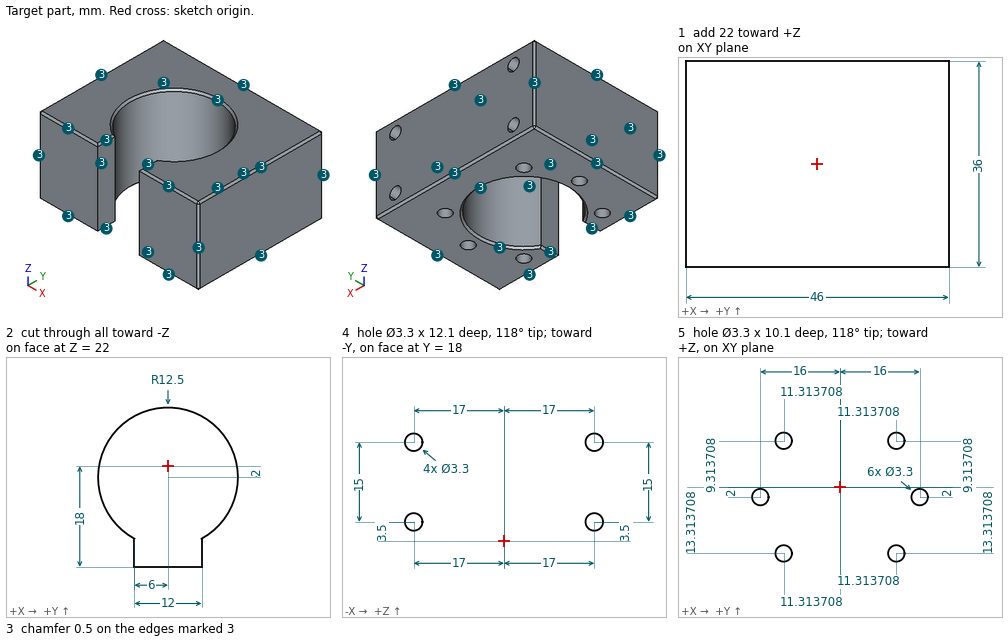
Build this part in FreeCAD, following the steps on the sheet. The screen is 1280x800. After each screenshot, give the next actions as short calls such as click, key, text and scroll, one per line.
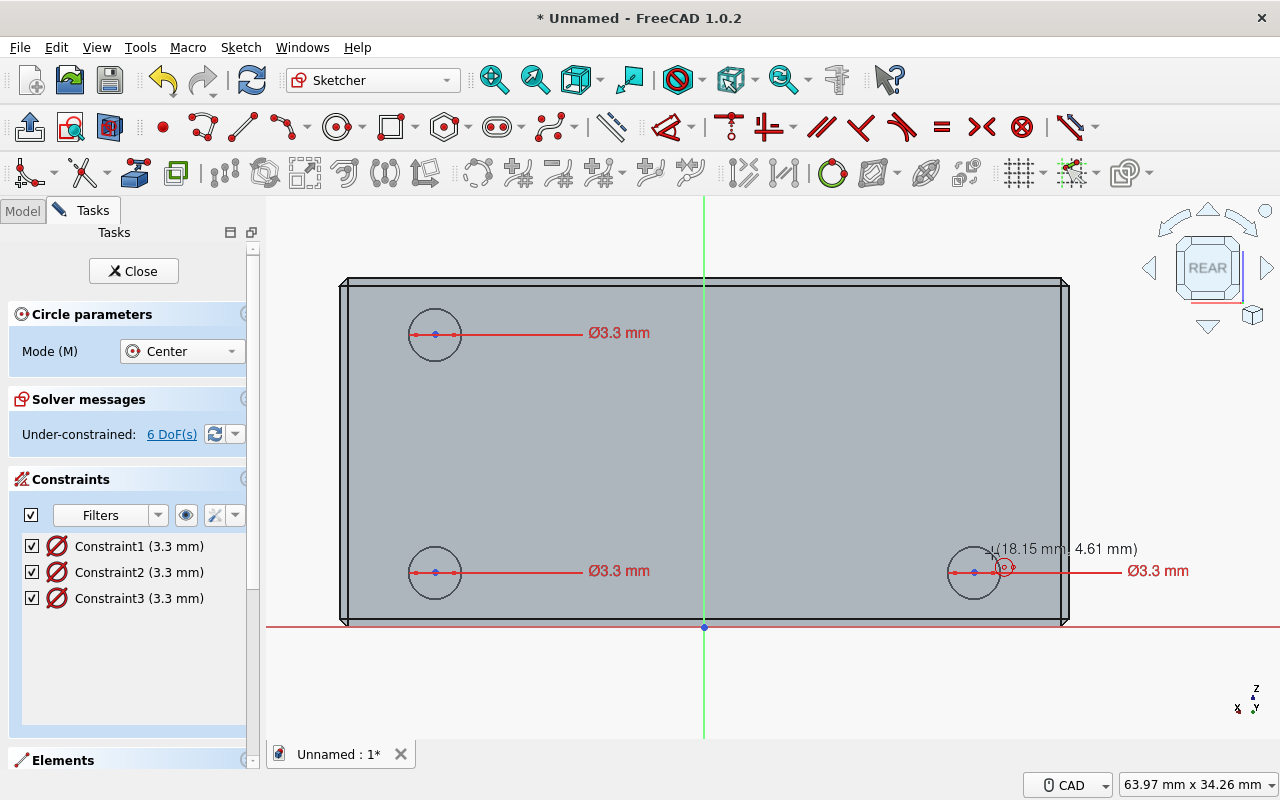
click(974, 334)
move(992, 315)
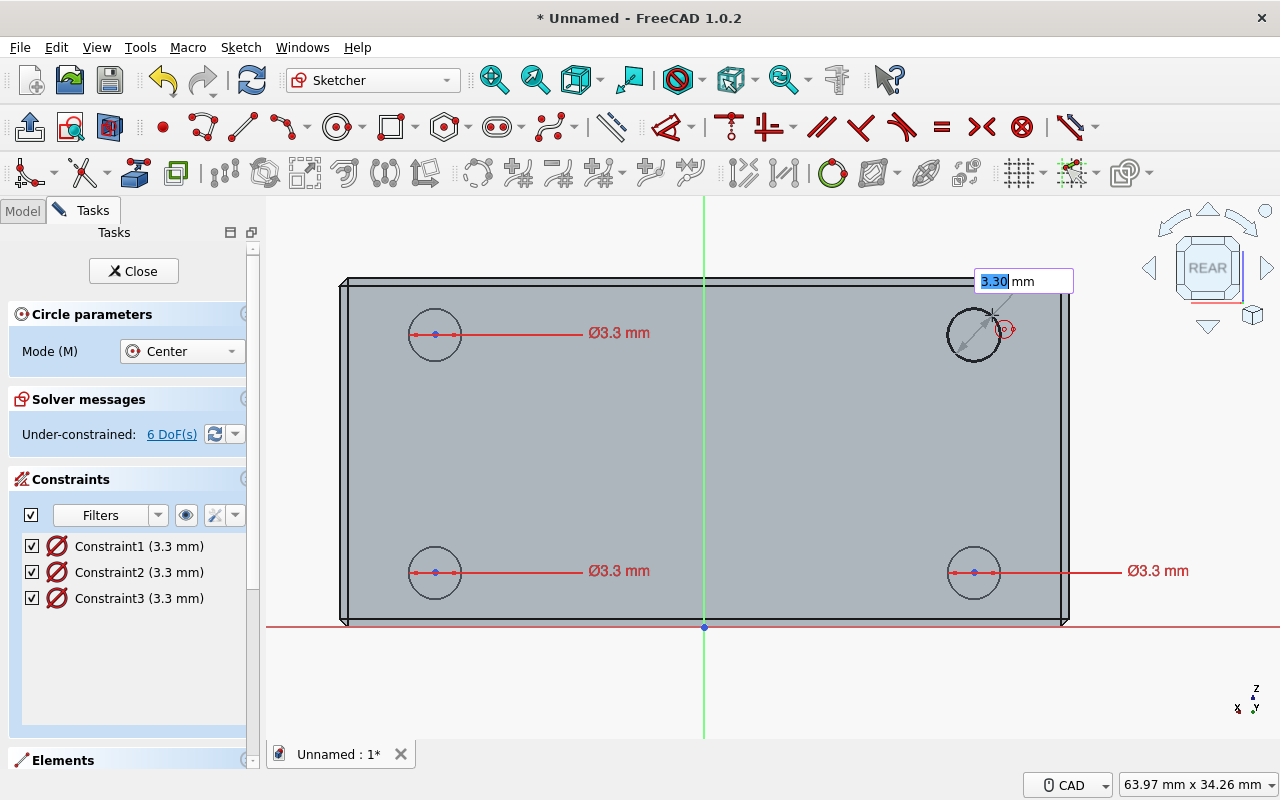
text(3.3)
key(Return)
key(Escape)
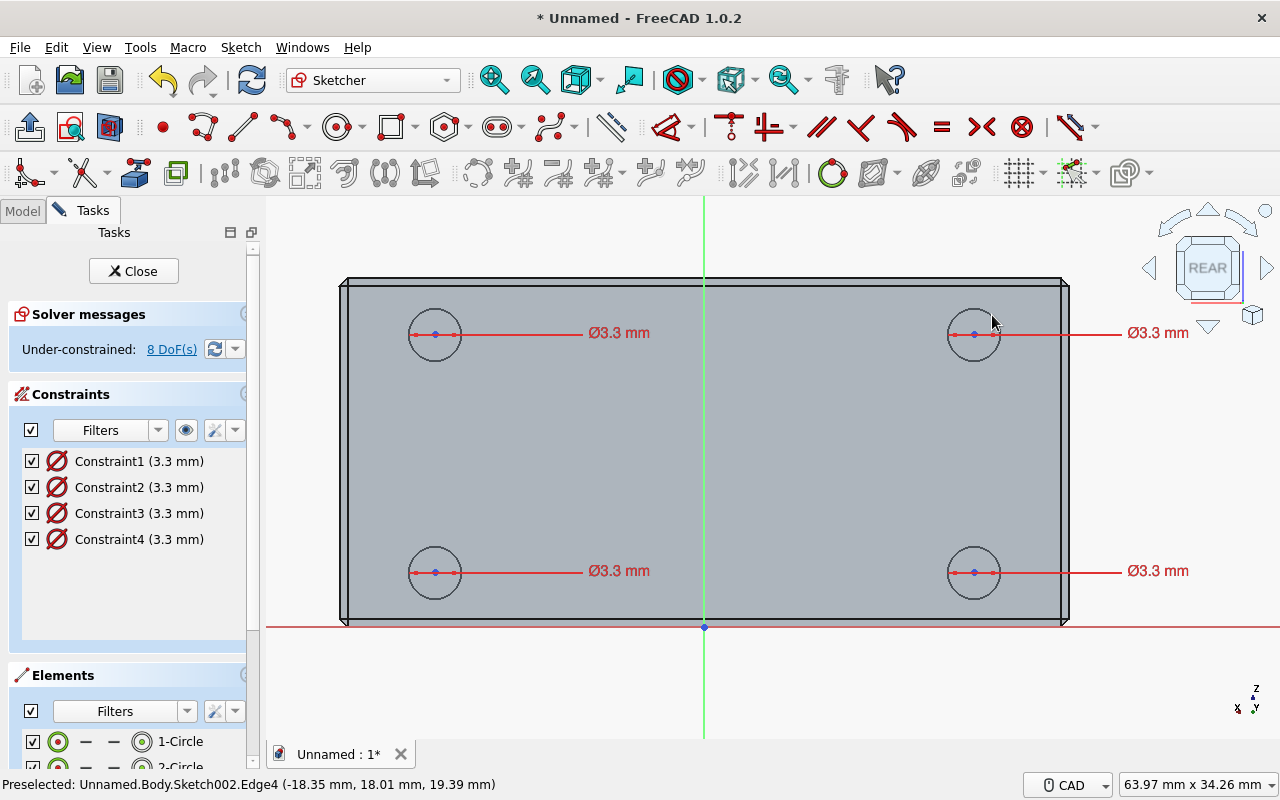
key(d)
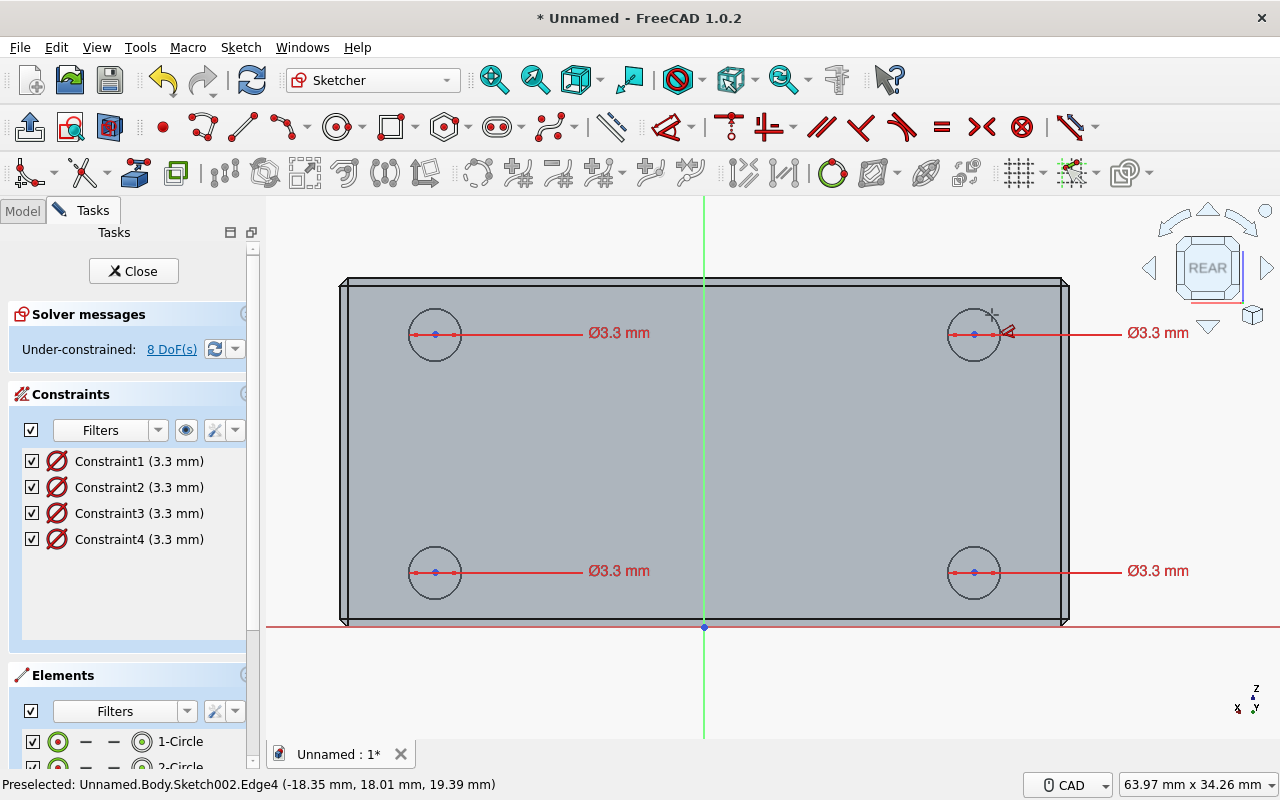
click(435, 335)
click(570, 661)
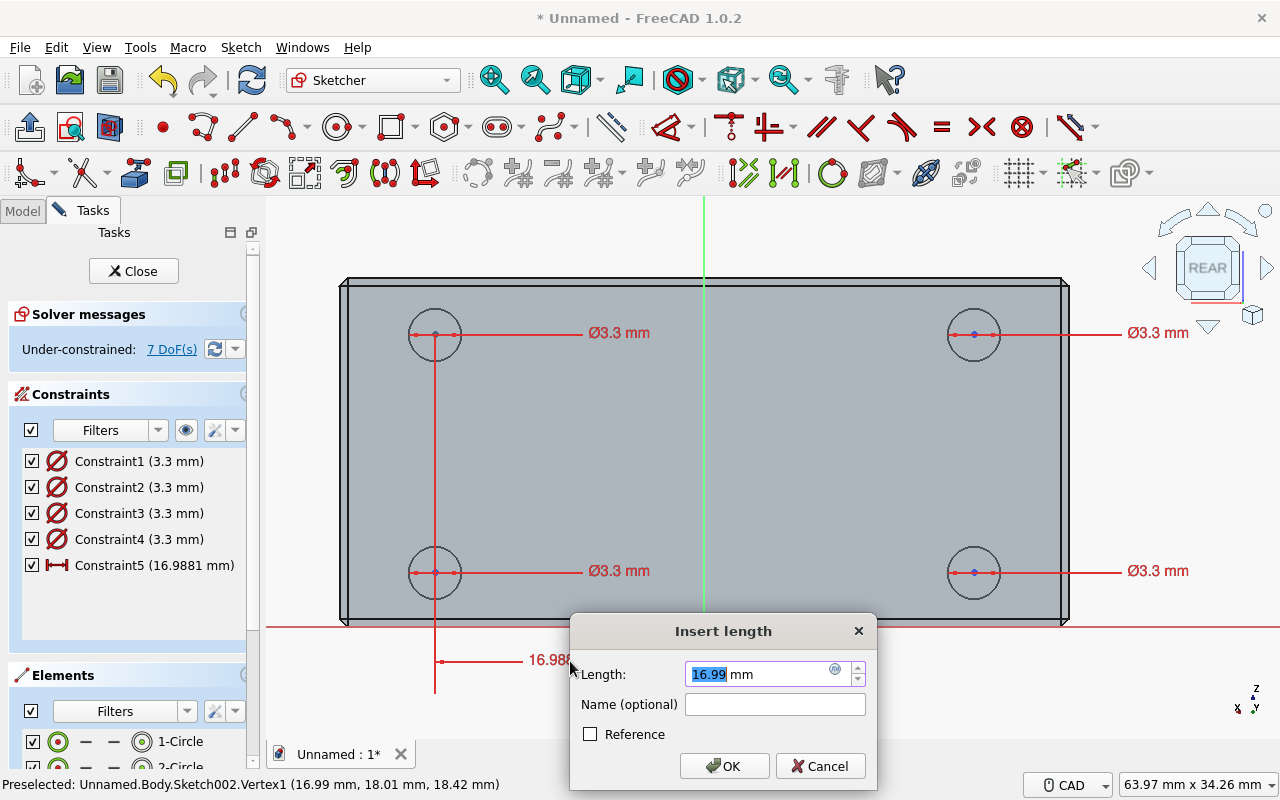
text(17)
key(Return)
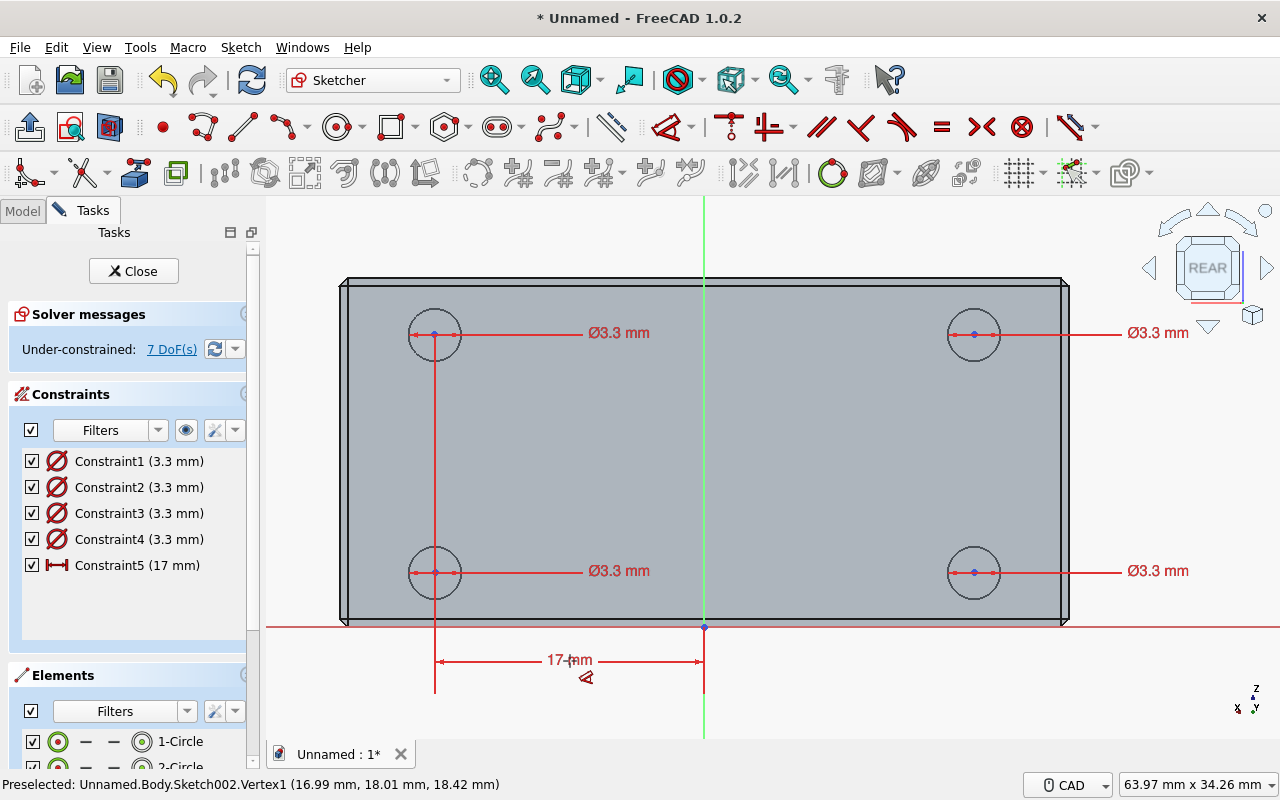
click(435, 573)
click(475, 661)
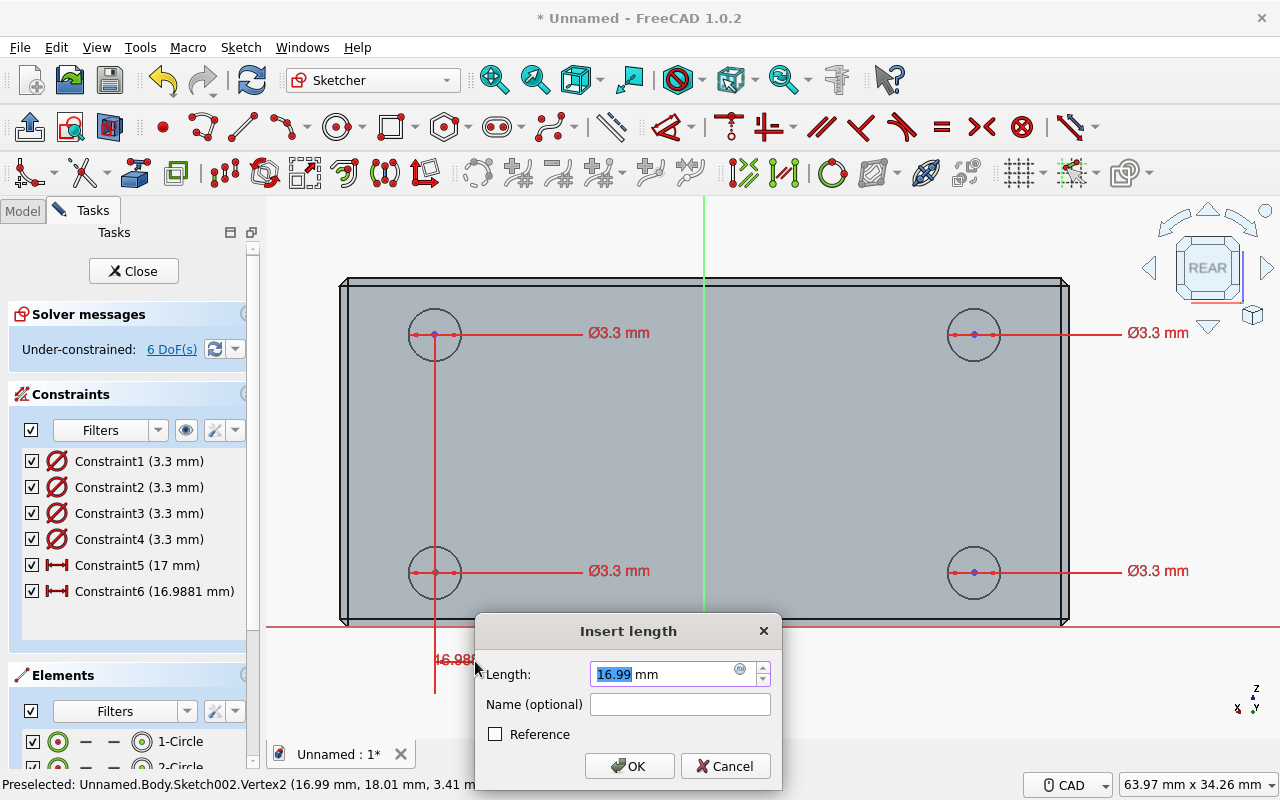
text(17)
key(Return)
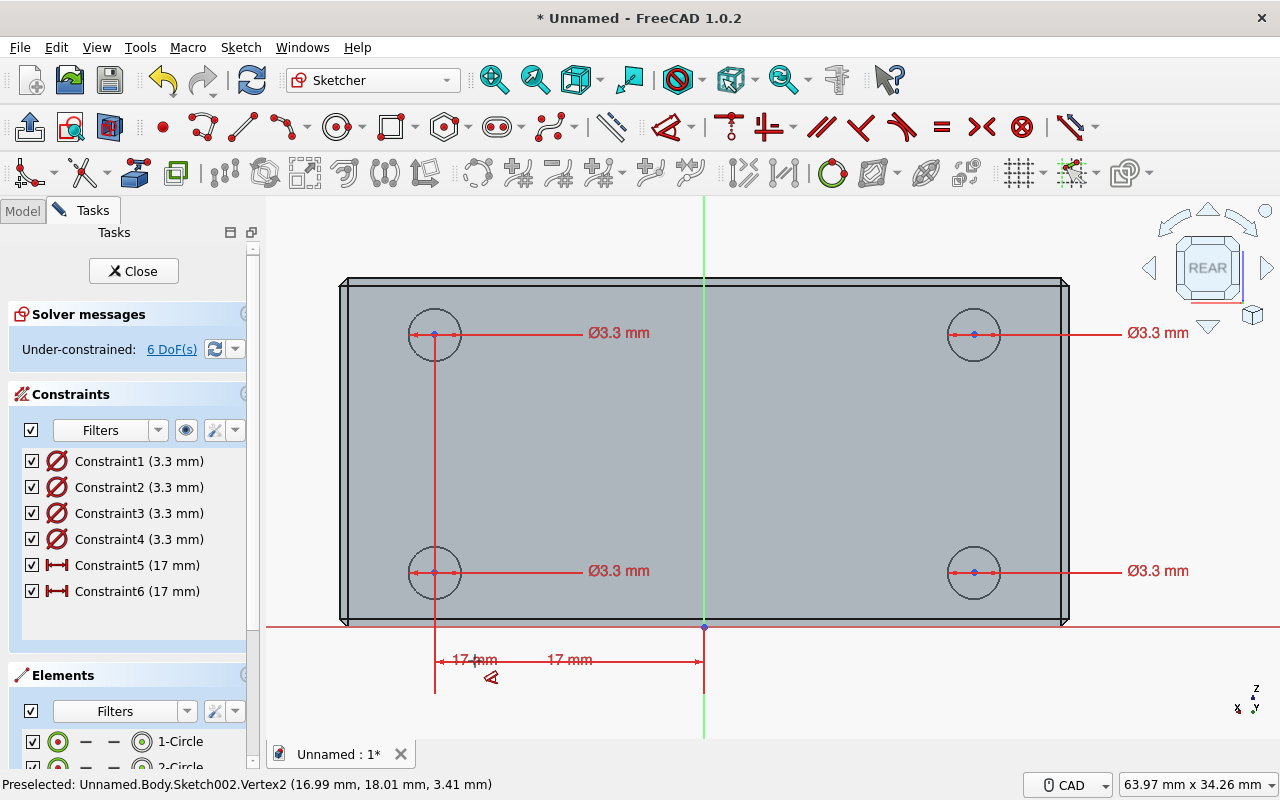
click(974, 573)
click(839, 661)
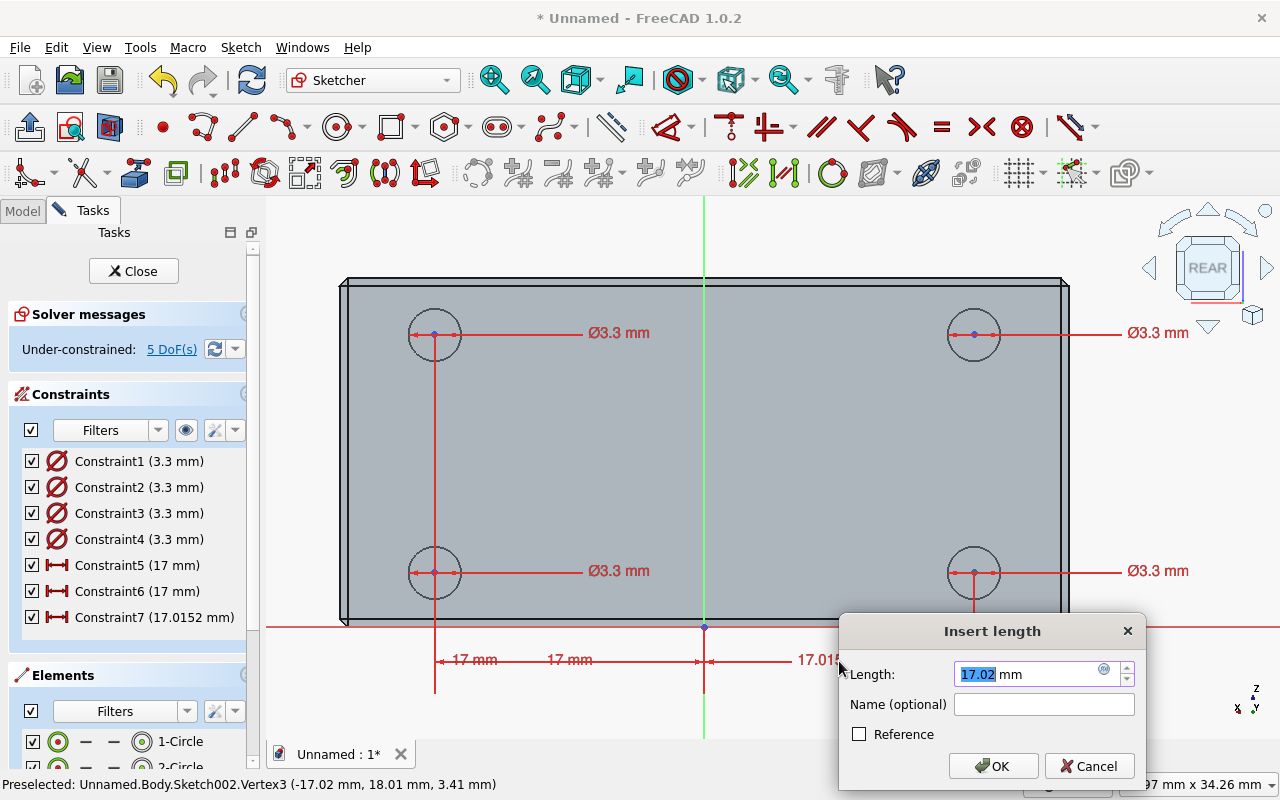
text(17)
key(Return)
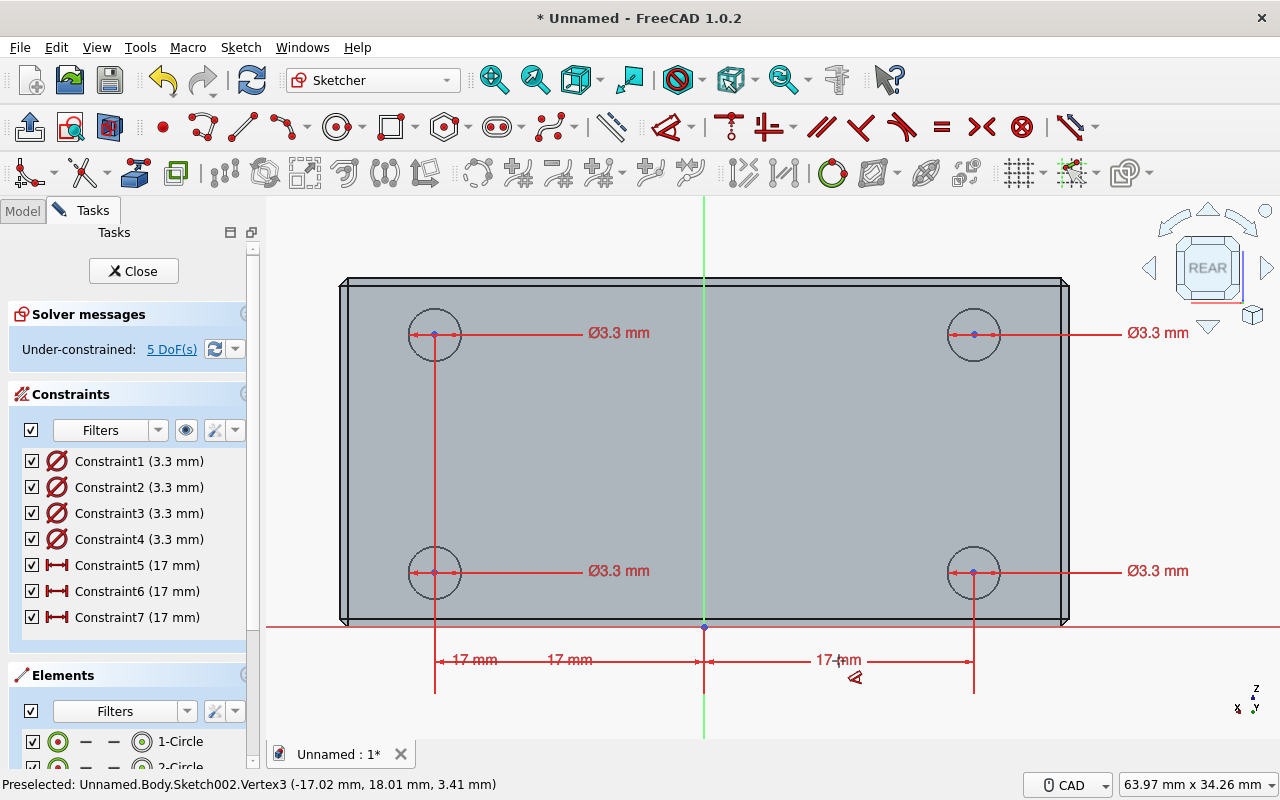
click(974, 335)
click(745, 661)